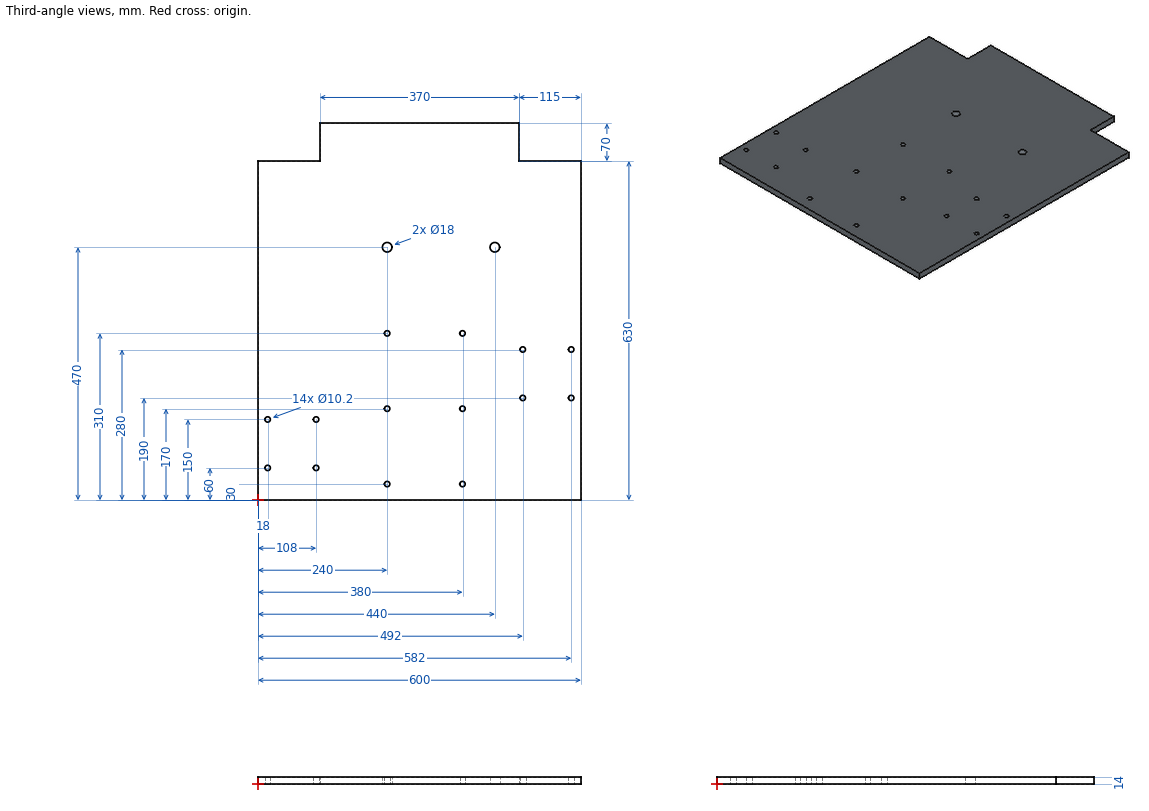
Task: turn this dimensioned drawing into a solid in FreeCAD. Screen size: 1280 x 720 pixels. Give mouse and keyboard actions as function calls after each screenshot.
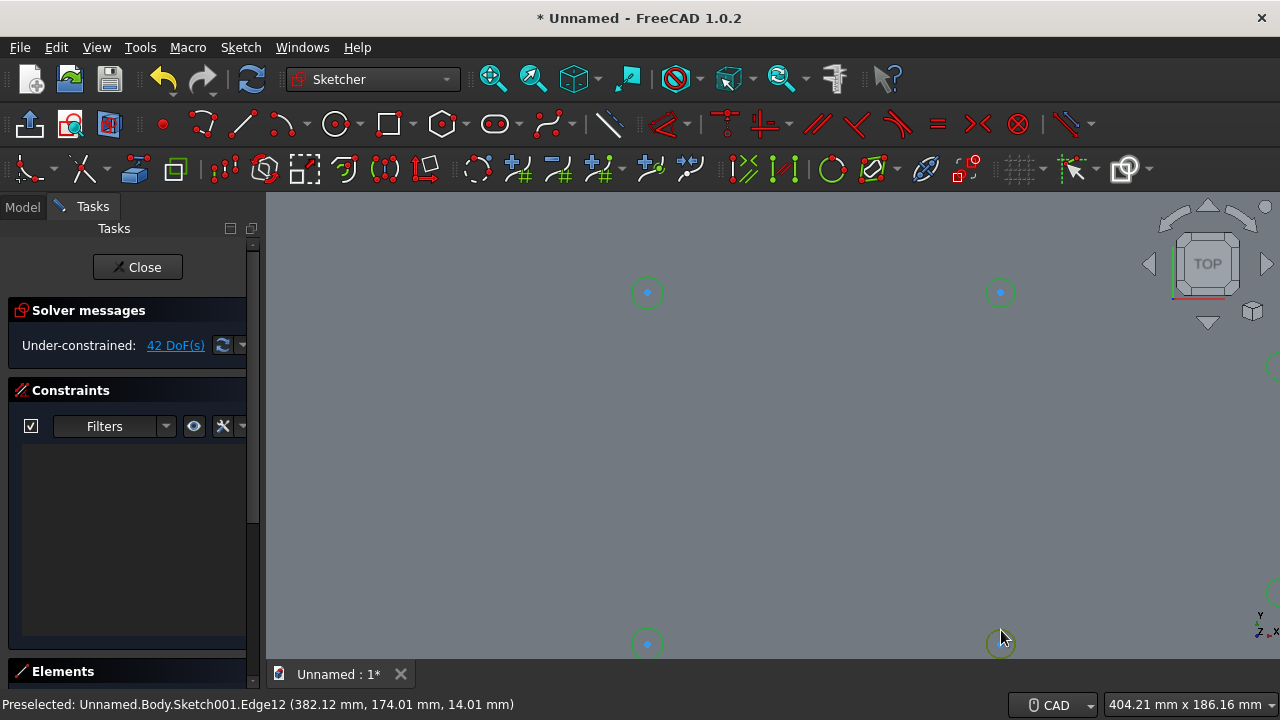
scroll(659, 282, down, 5)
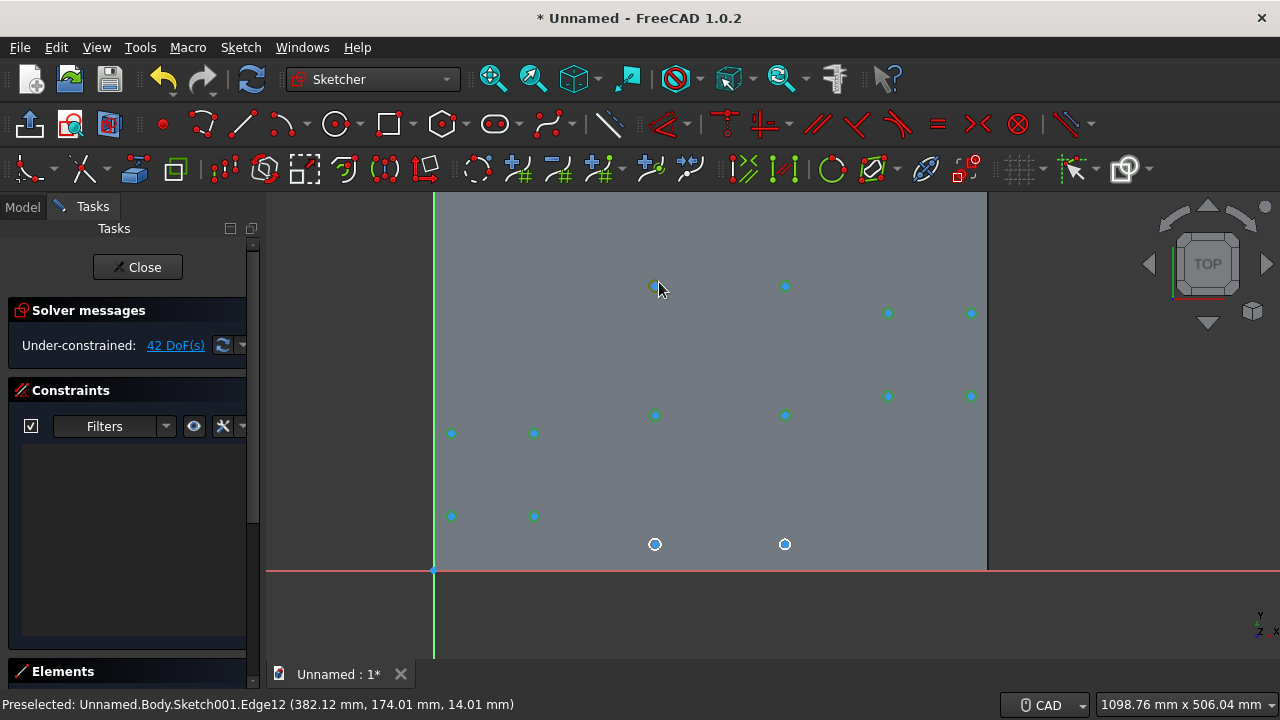
scroll(659, 540, up, 5)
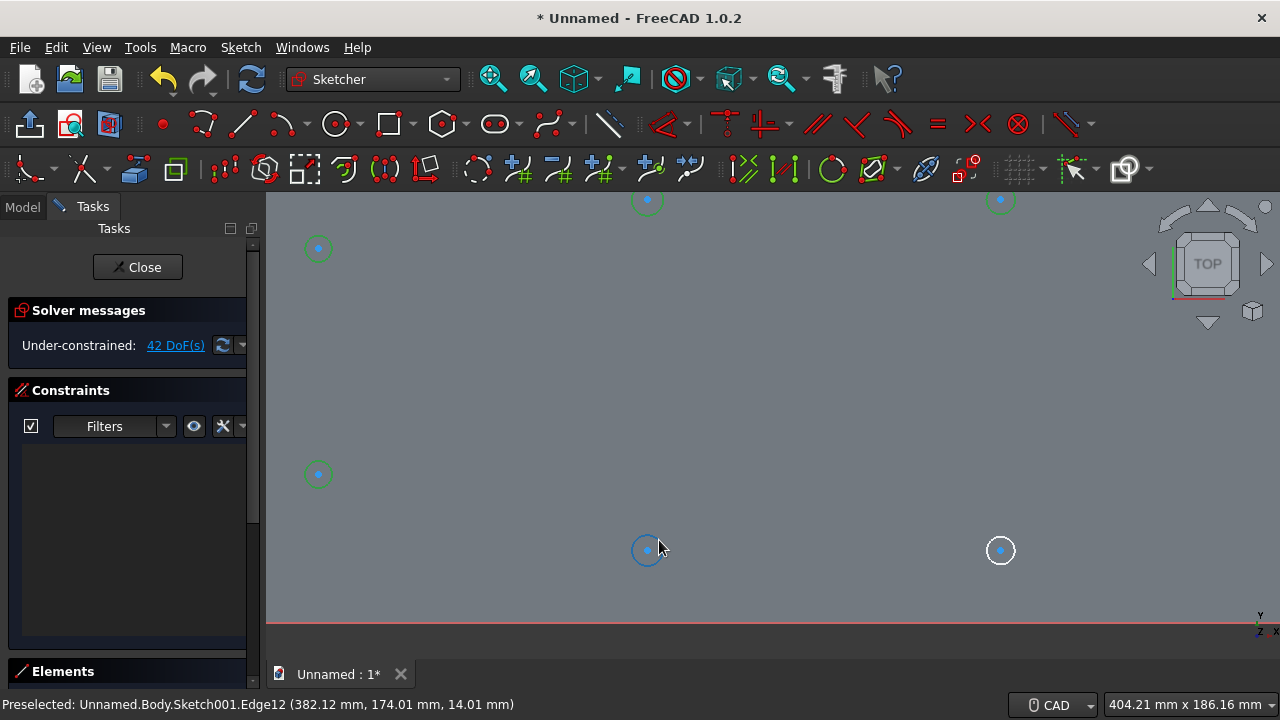
click(658, 540)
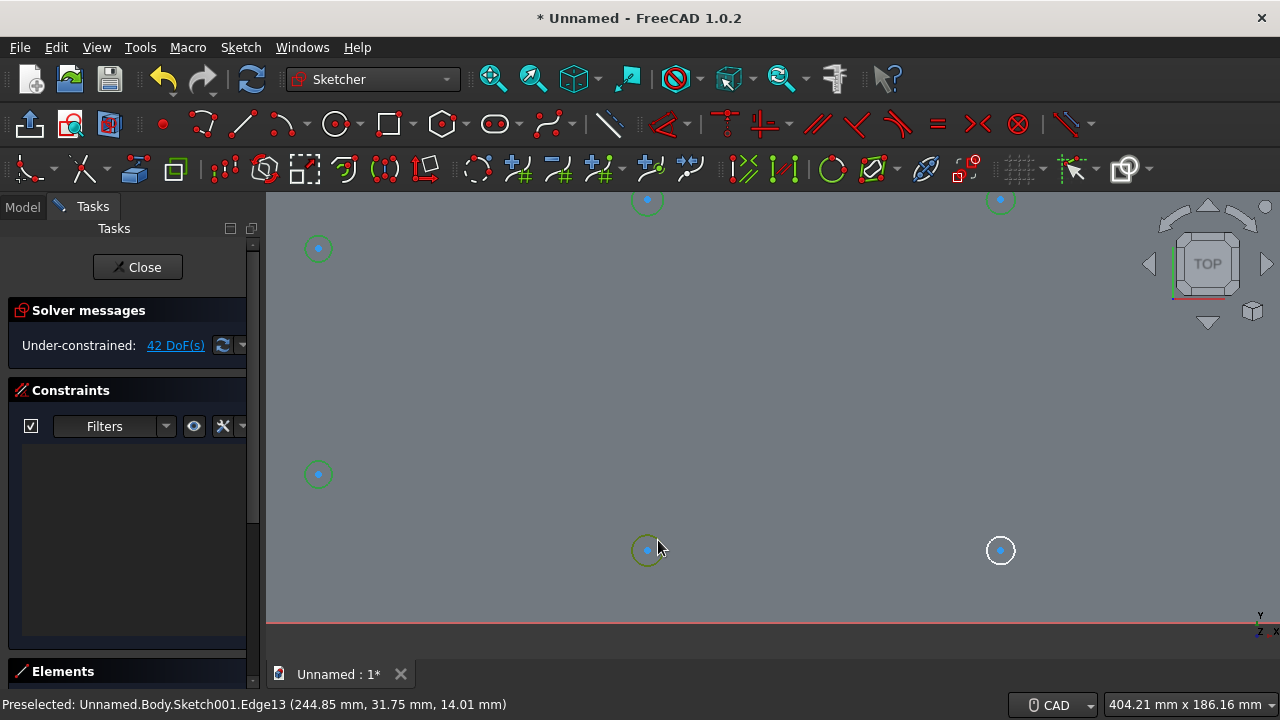
click(1011, 541)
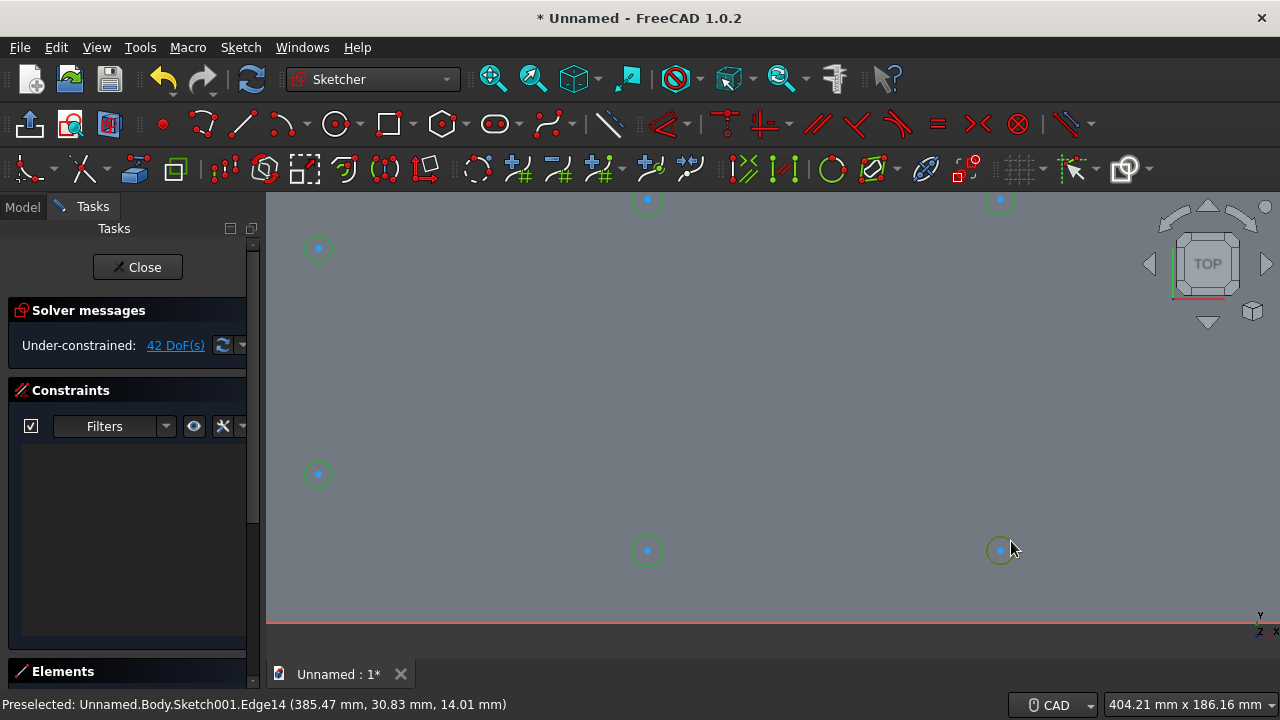
key(e)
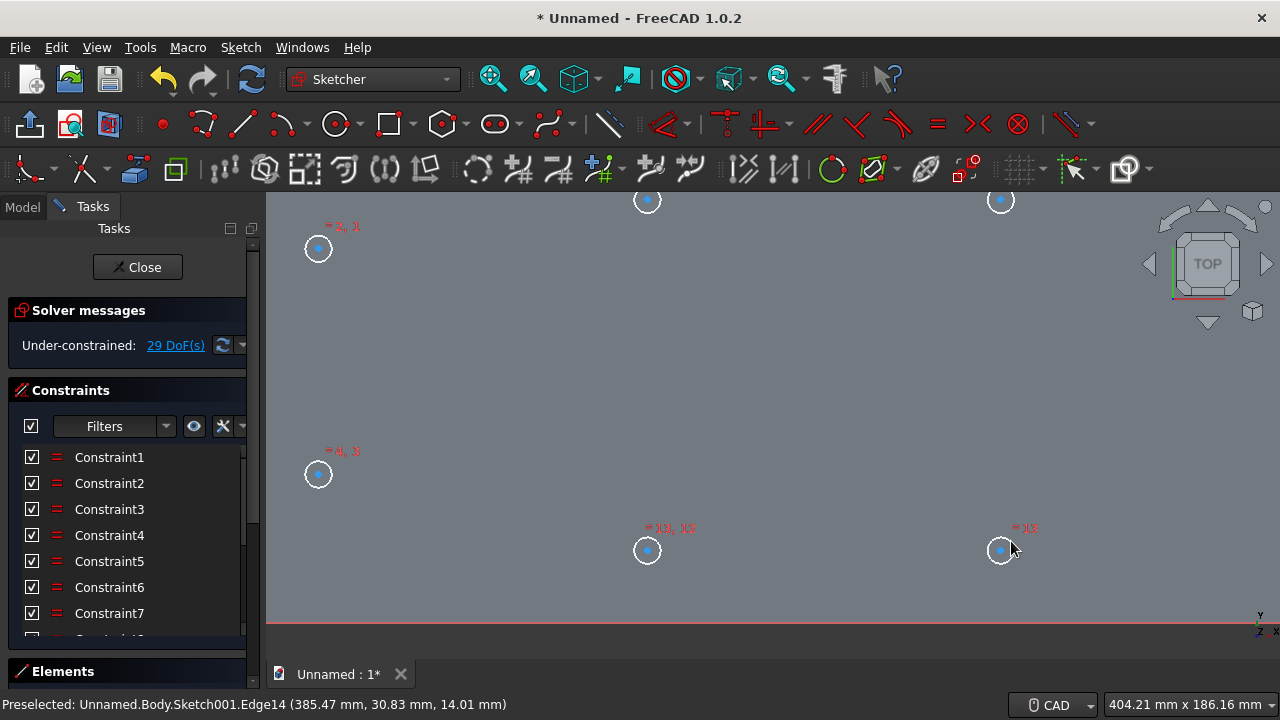
key(d)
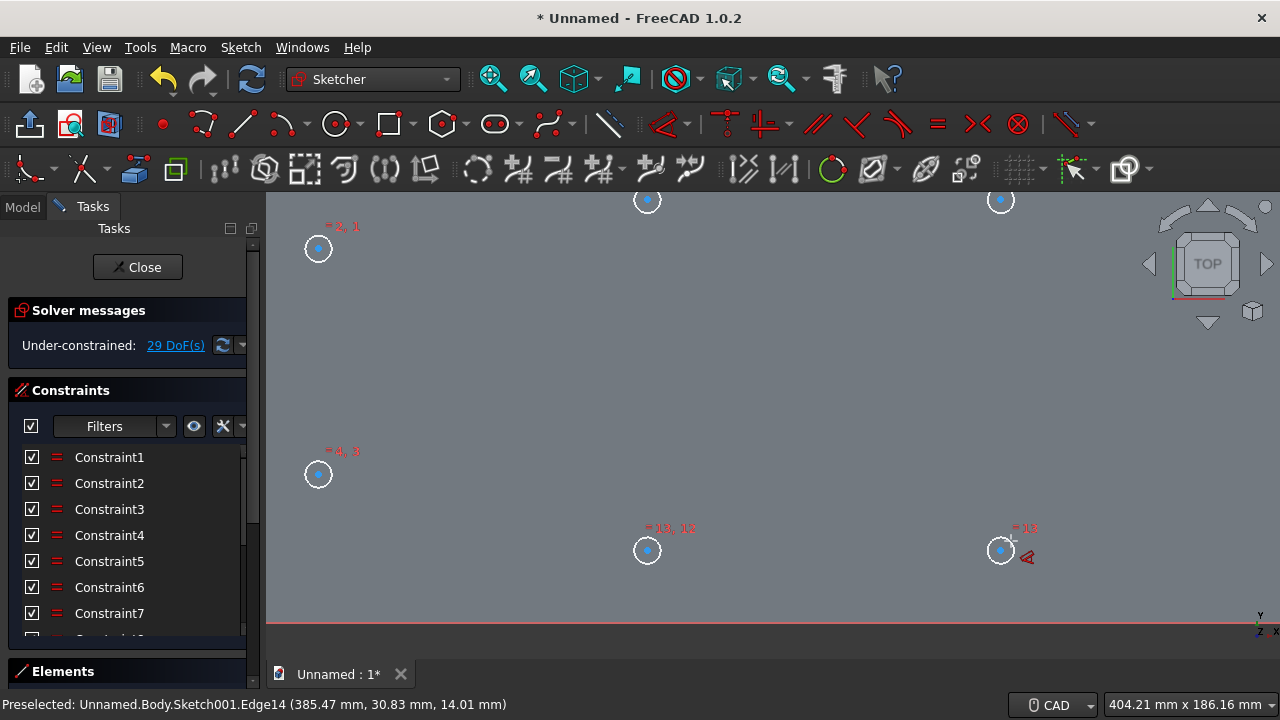
scroll(659, 541, down, 5)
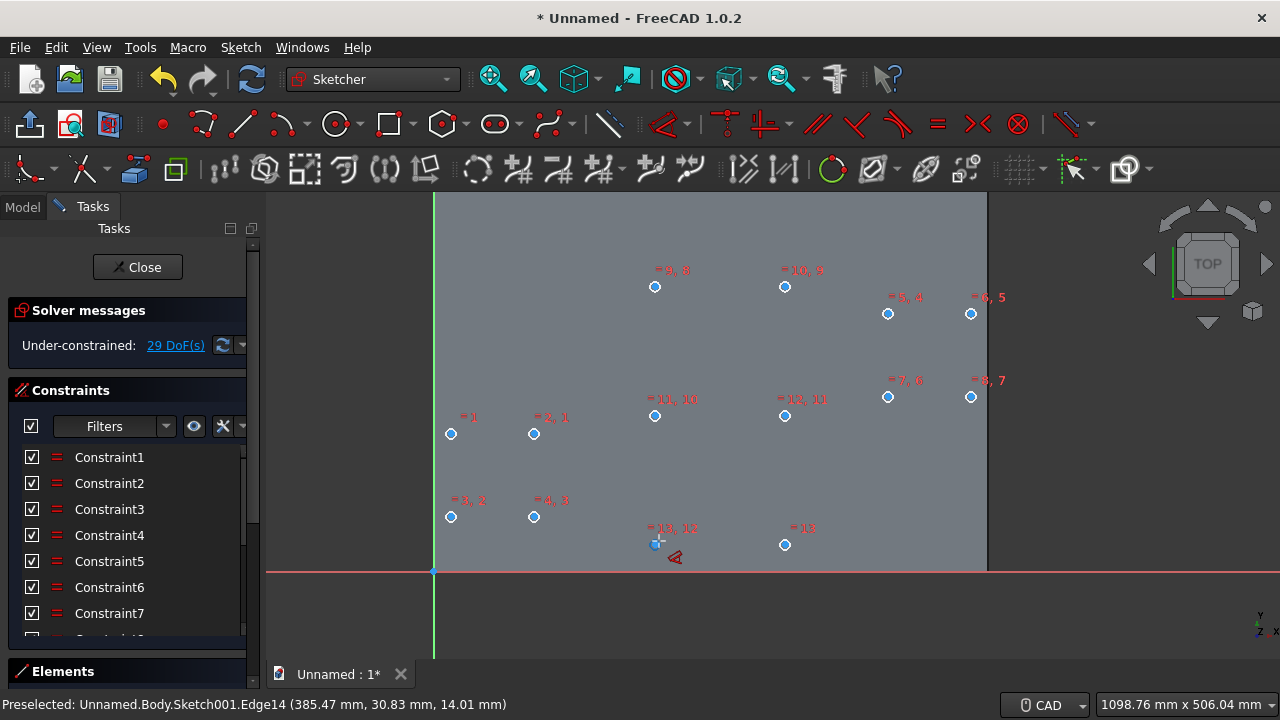
scroll(454, 431, up, 8)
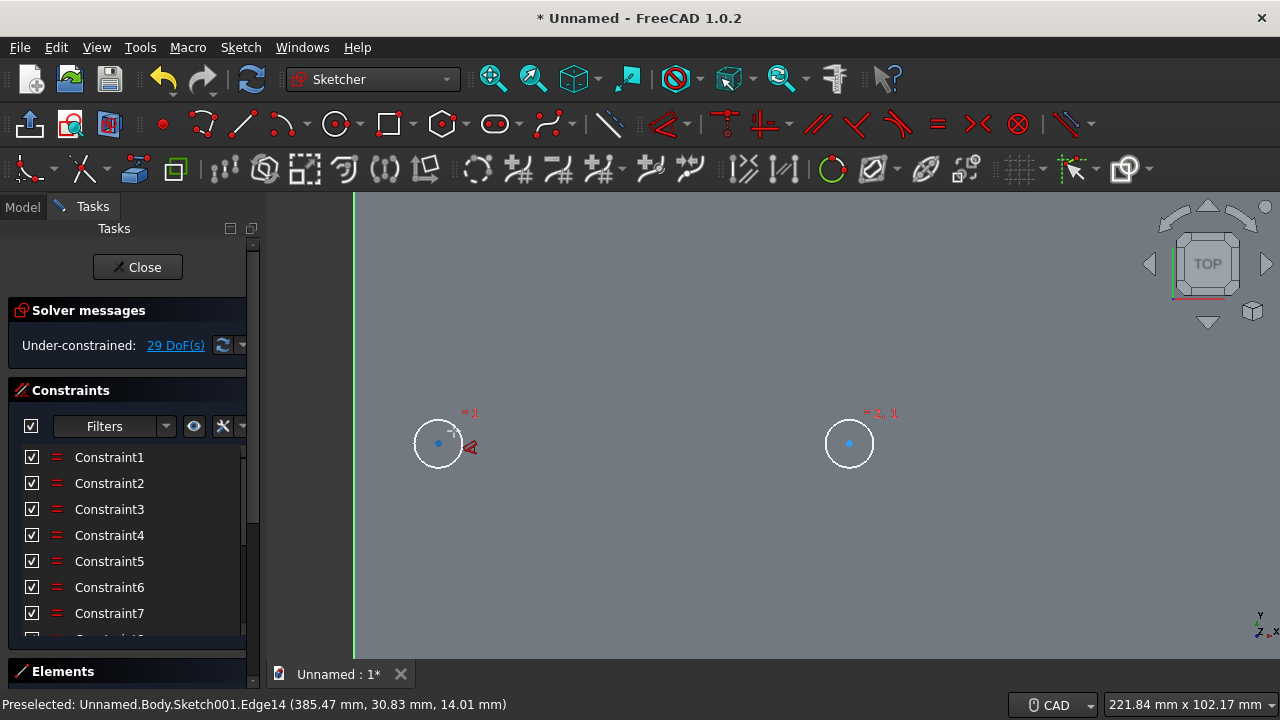
click(455, 427)
click(477, 404)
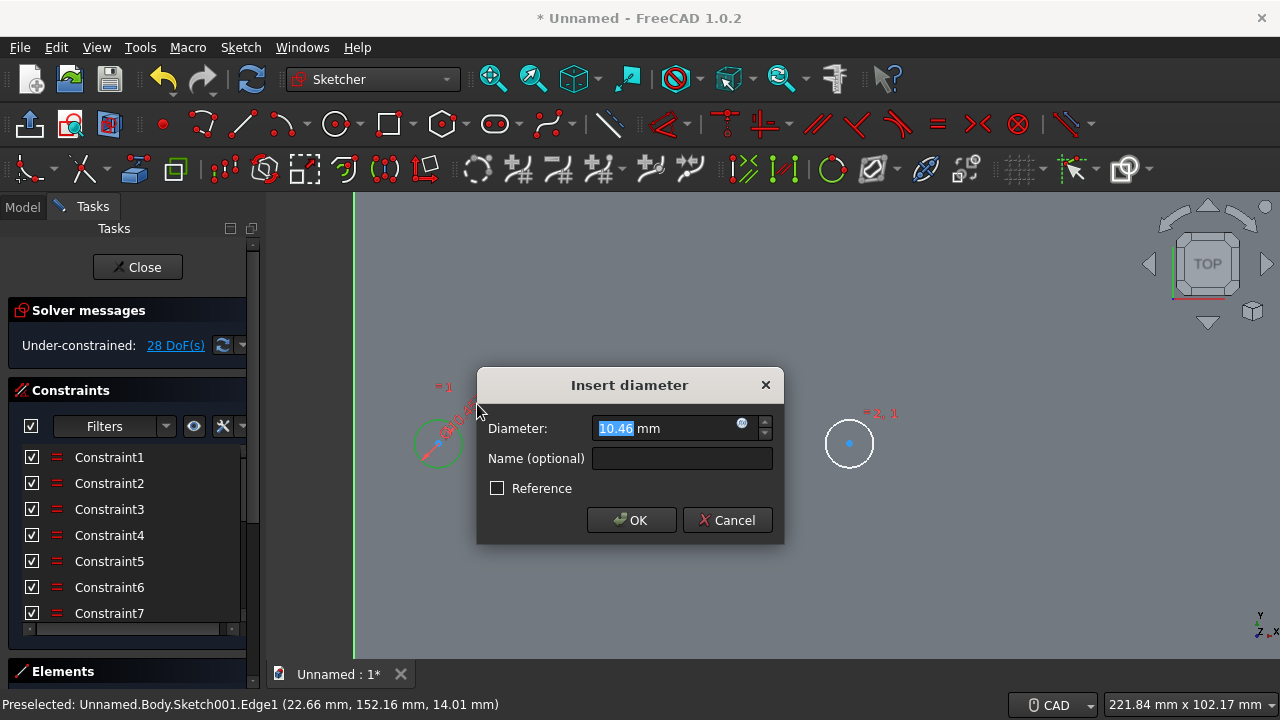
text(10.2)
key(Return)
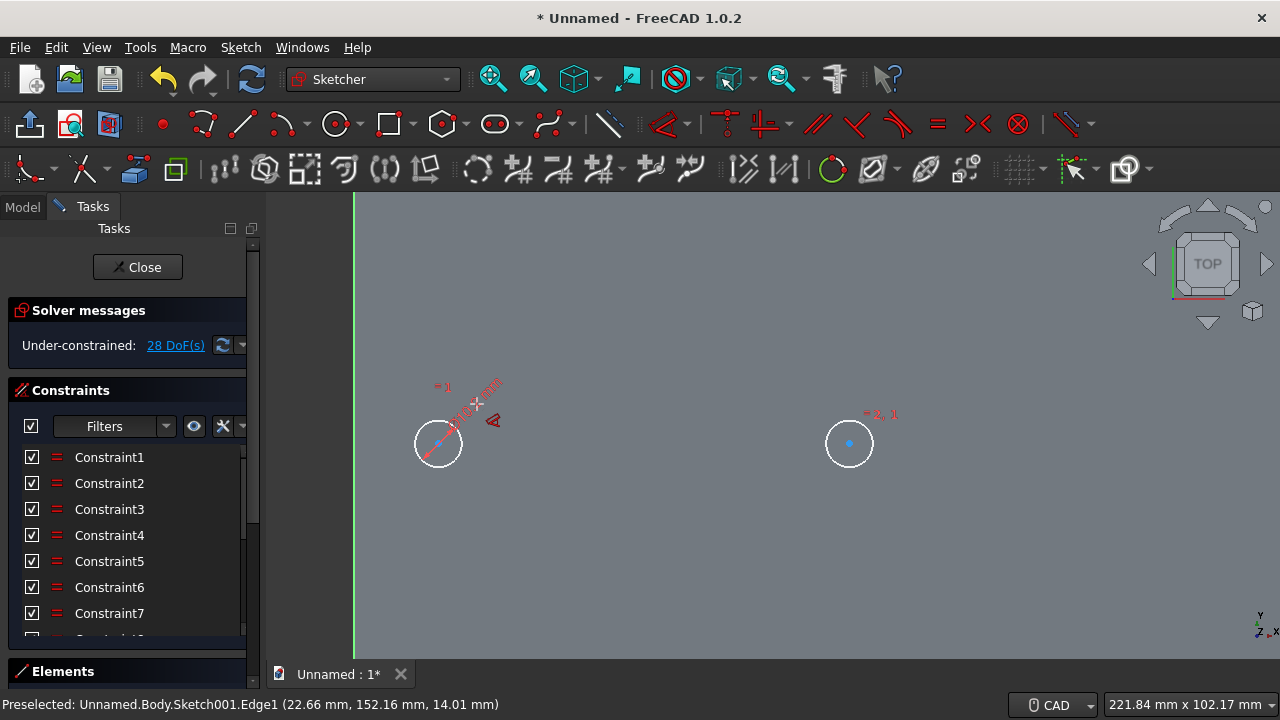
click(438, 444)
click(396, 410)